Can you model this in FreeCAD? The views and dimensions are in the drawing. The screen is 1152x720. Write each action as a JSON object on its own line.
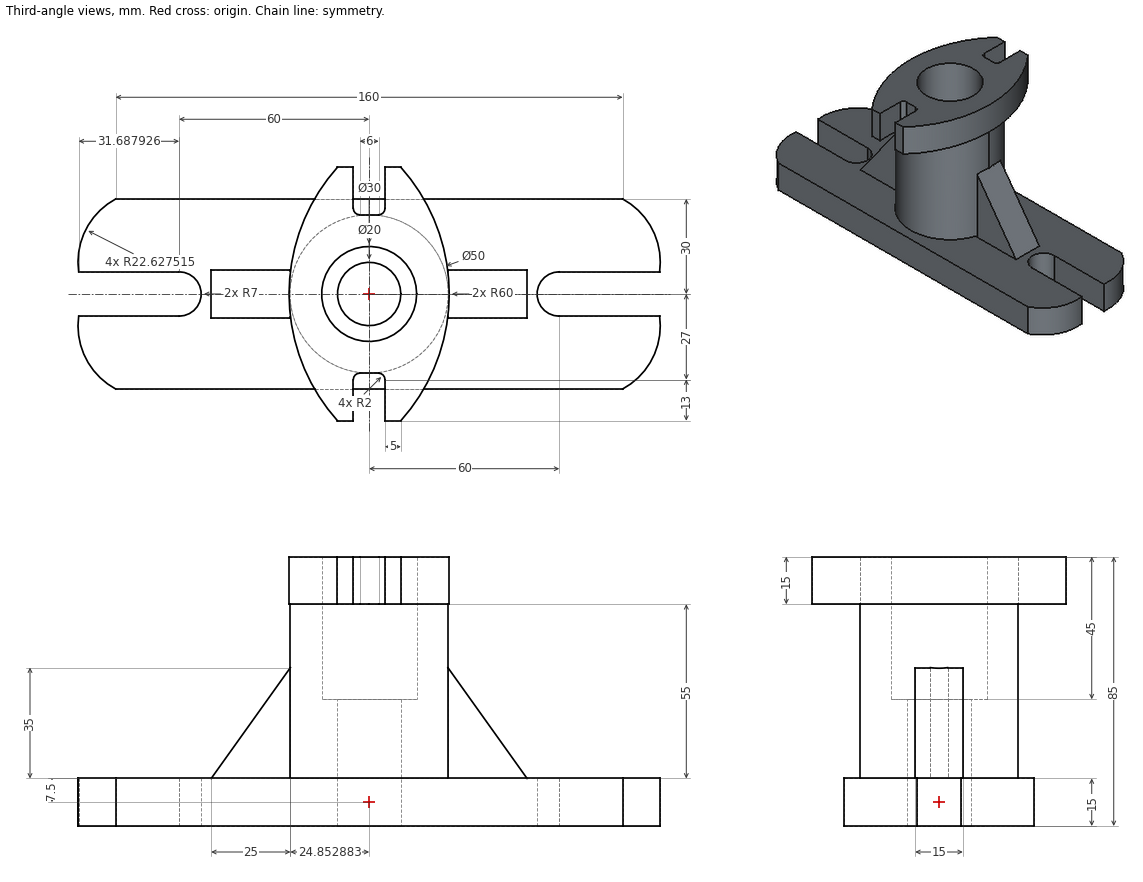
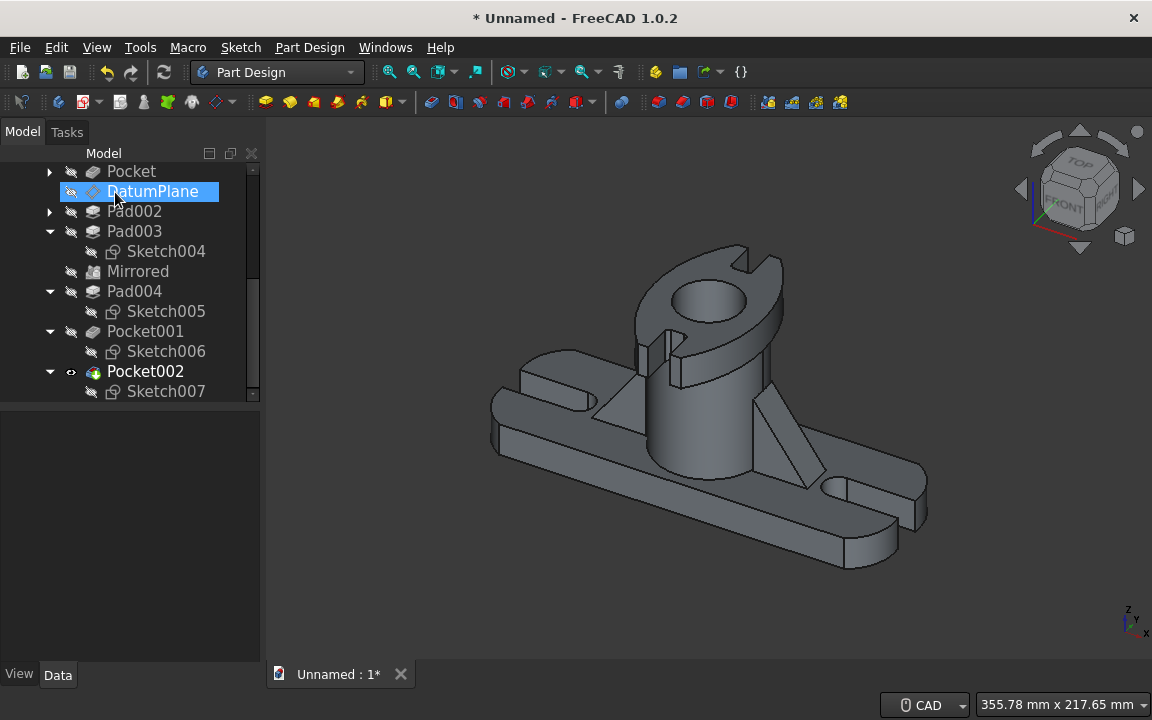
{"action": "key", "text": "0"}